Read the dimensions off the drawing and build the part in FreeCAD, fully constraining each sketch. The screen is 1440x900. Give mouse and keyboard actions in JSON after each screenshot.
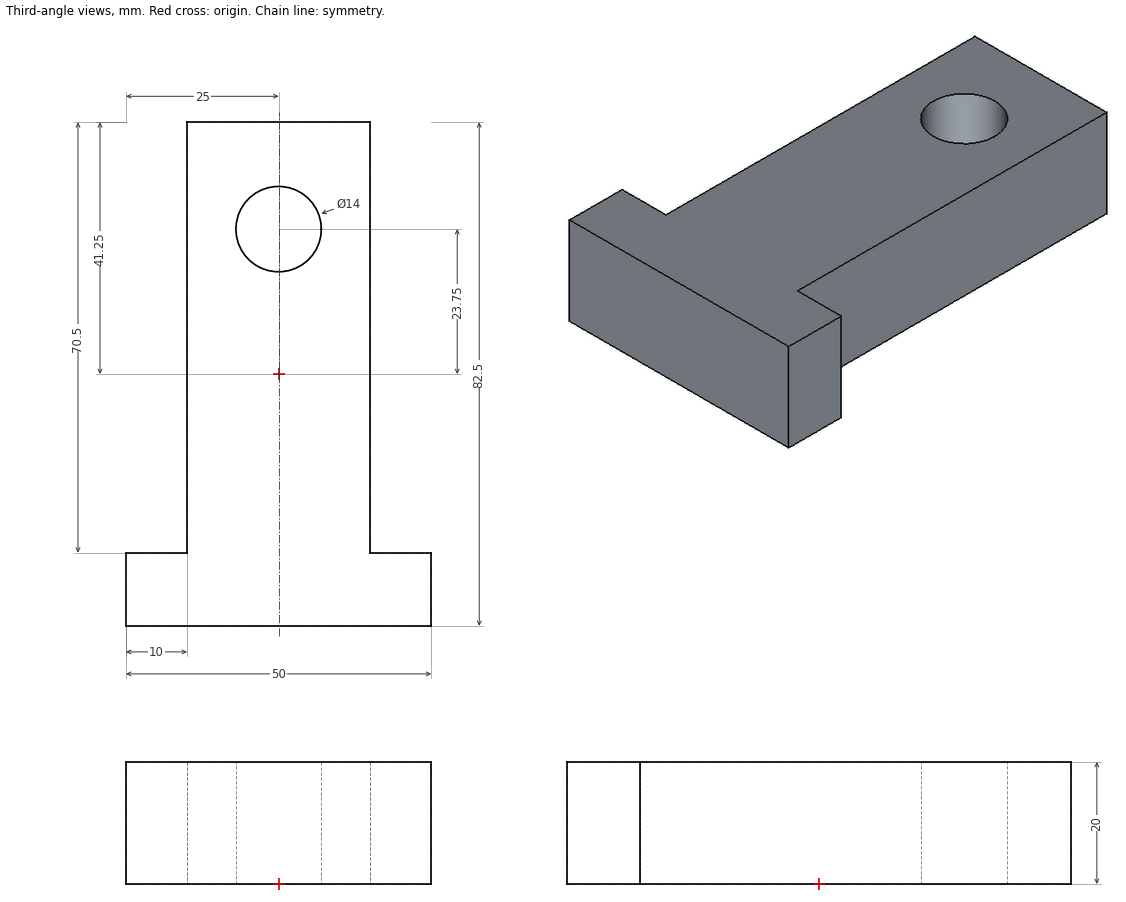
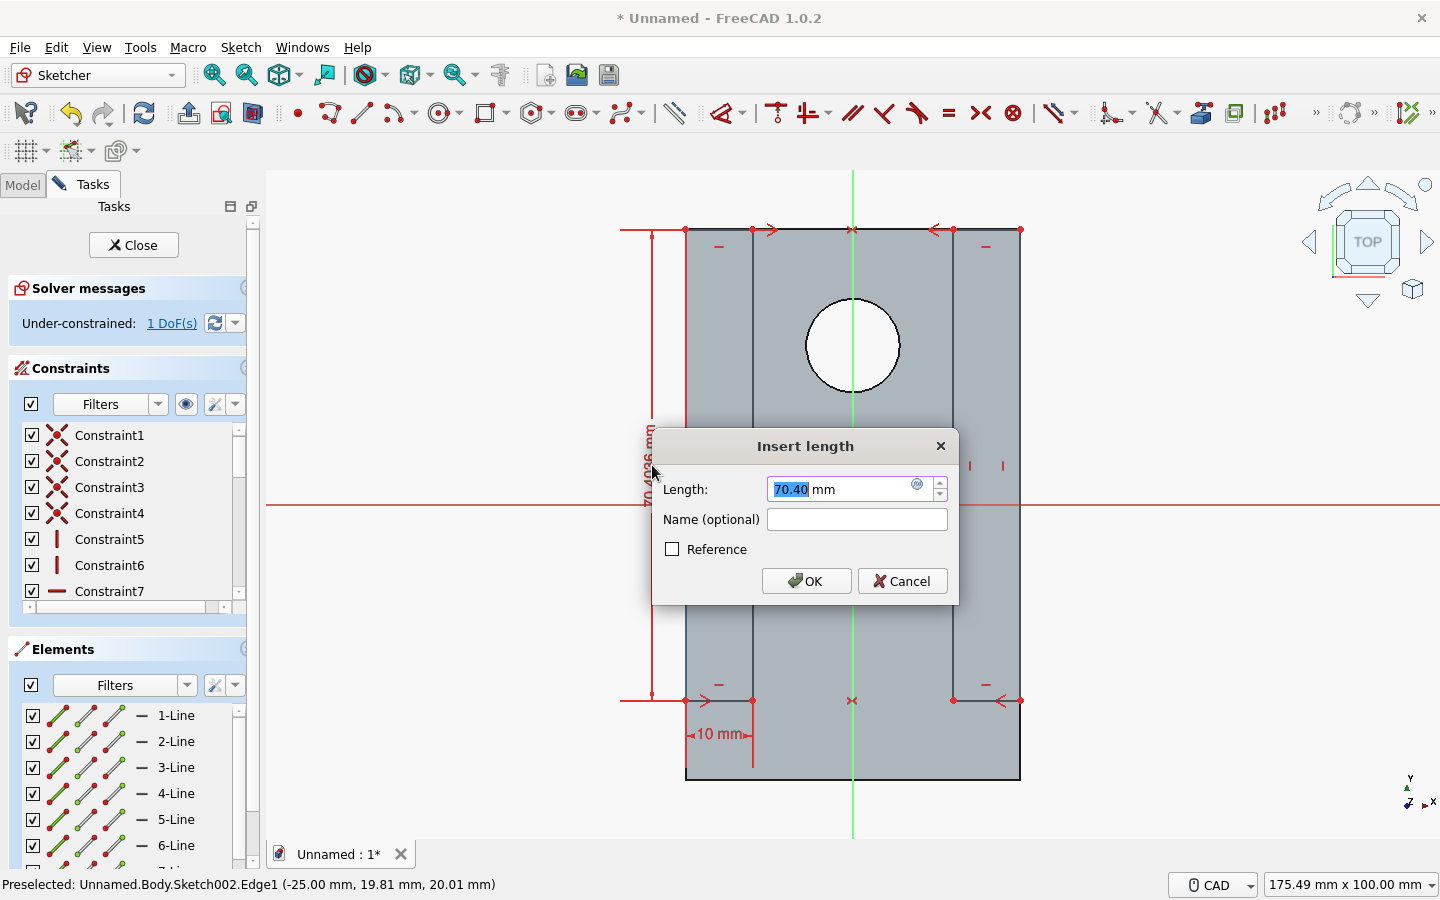
{"action": "type", "text": "70.5"}
{"action": "key", "text": "Return"}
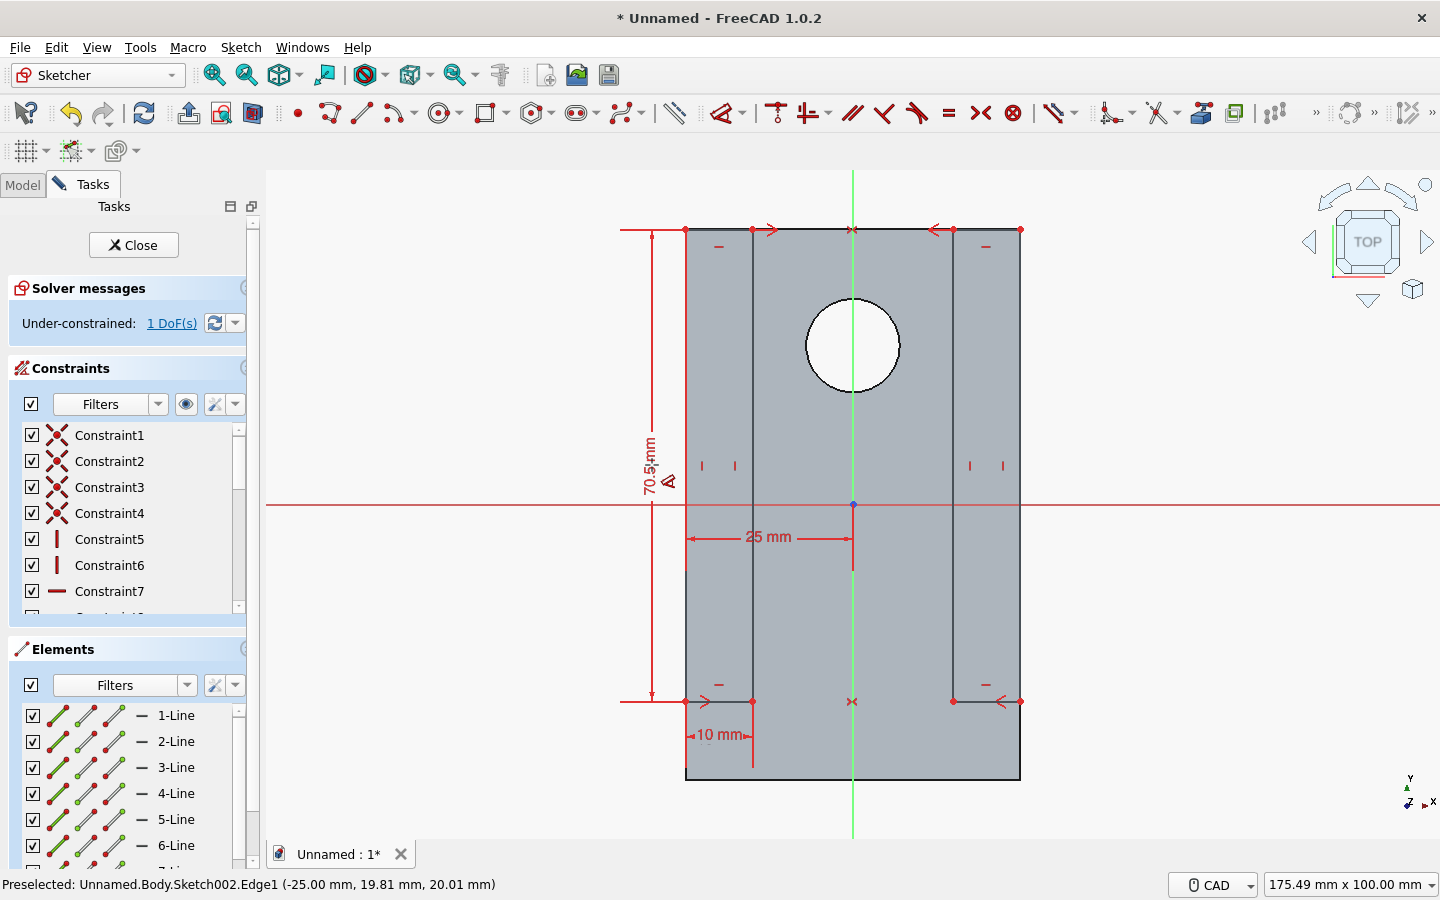
{"action": "left_click", "coordinate": [686, 230]}
{"action": "left_click", "coordinate": [652, 367]}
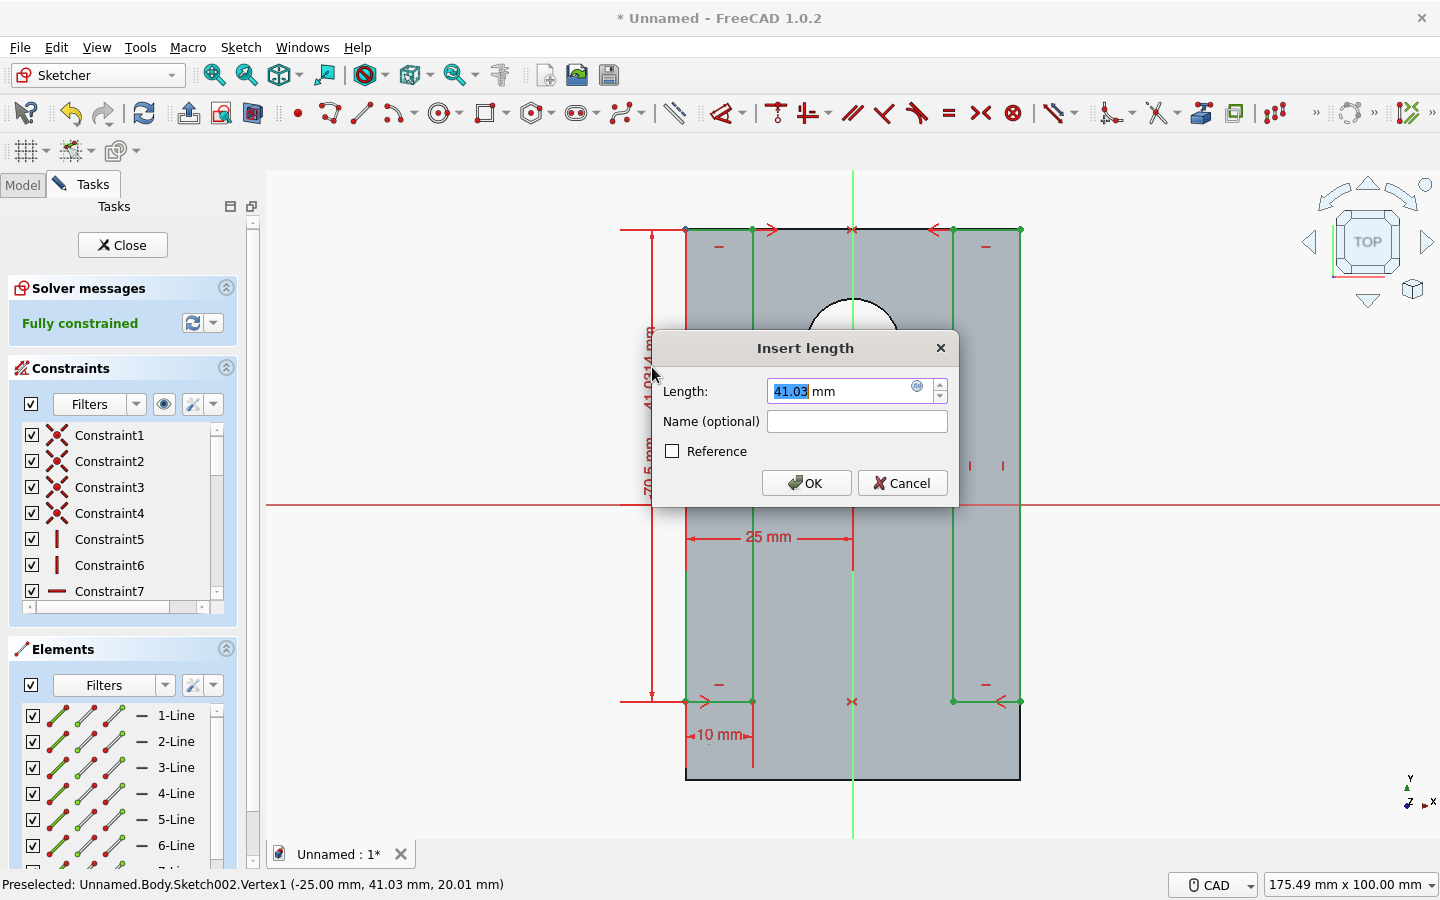
{"action": "type", "text": "41.25"}
{"action": "key", "text": "Return"}
{"action": "key", "text": "Escape"}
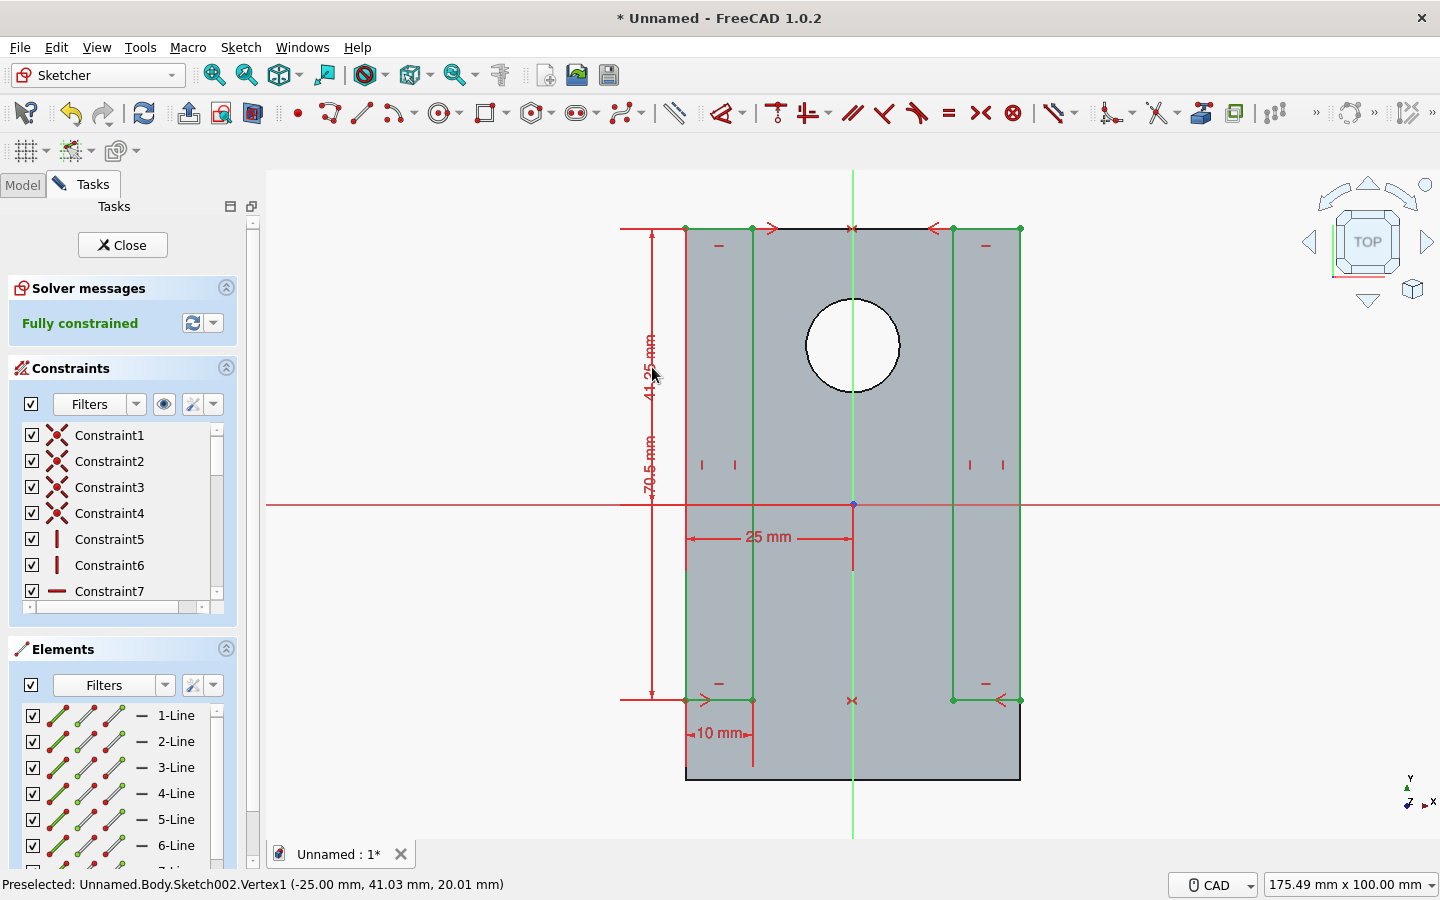
{"action": "left_click", "coordinate": [123, 245]}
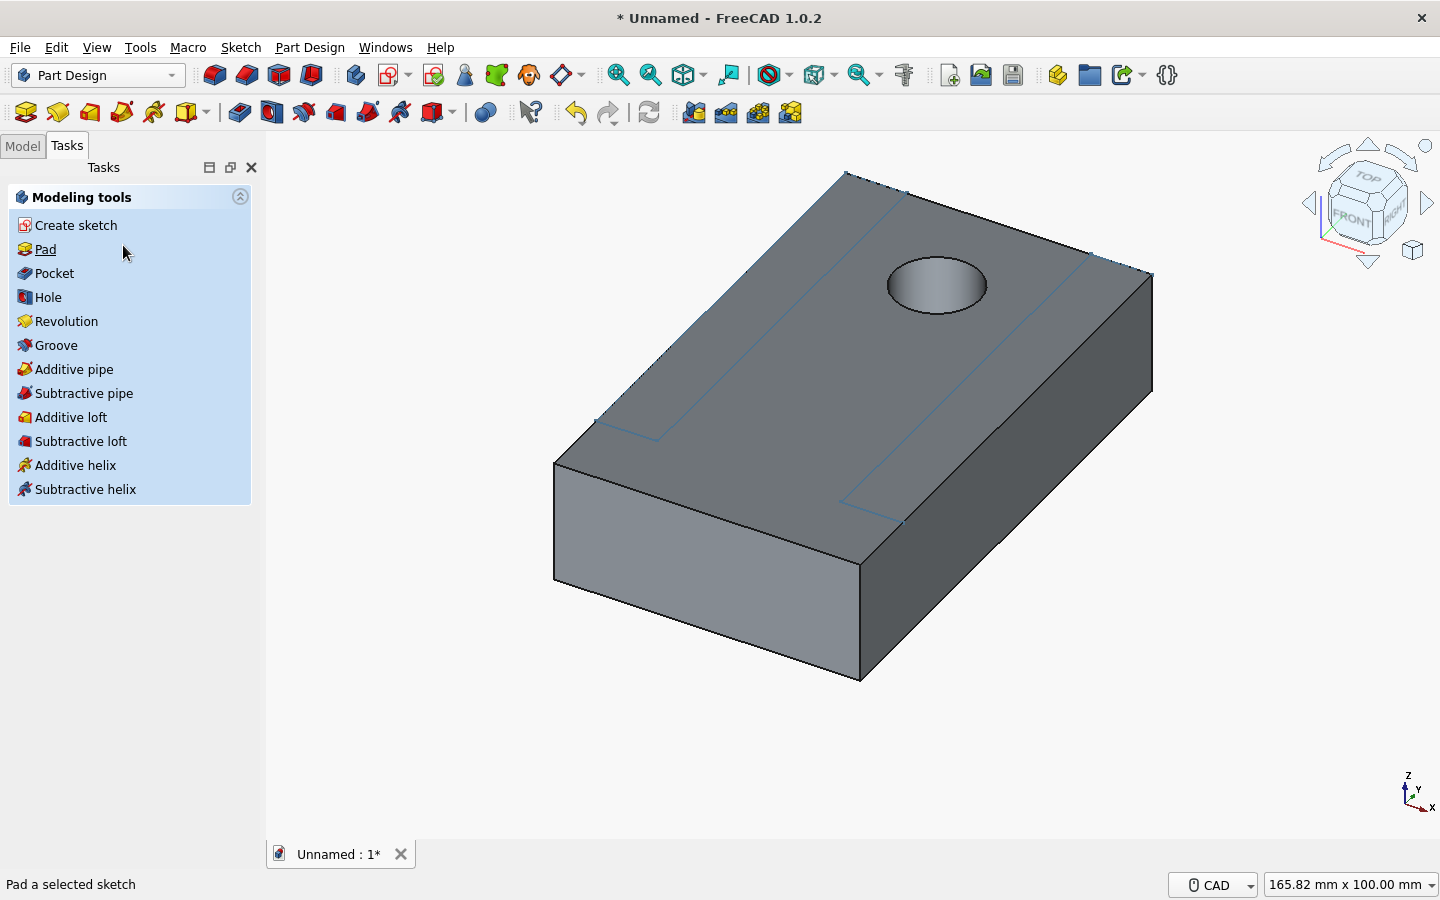
{"action": "left_click", "coordinate": [240, 112]}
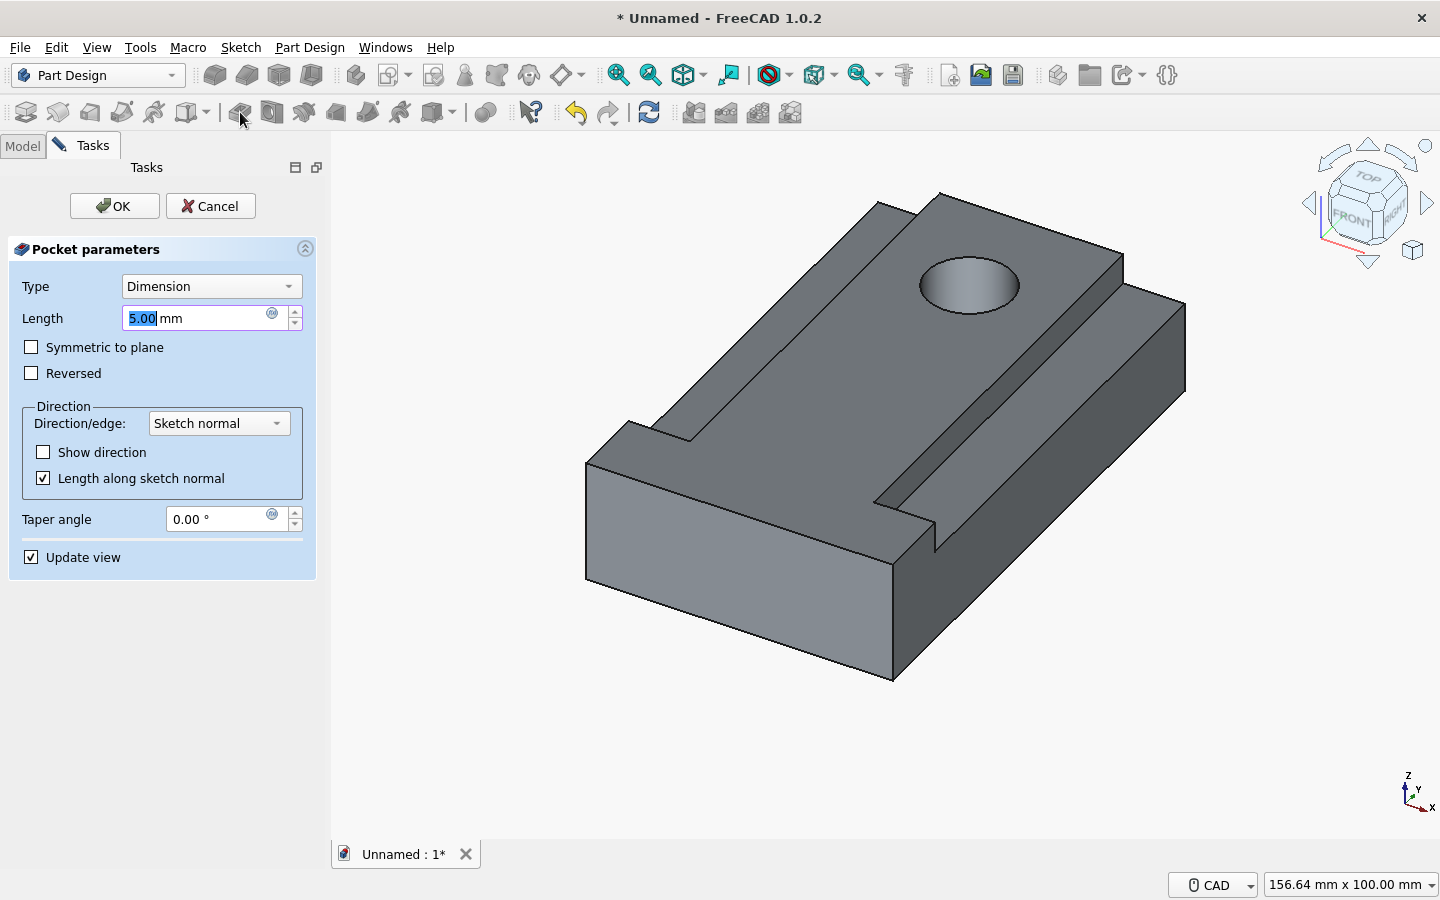
{"action": "left_click", "coordinate": [212, 286]}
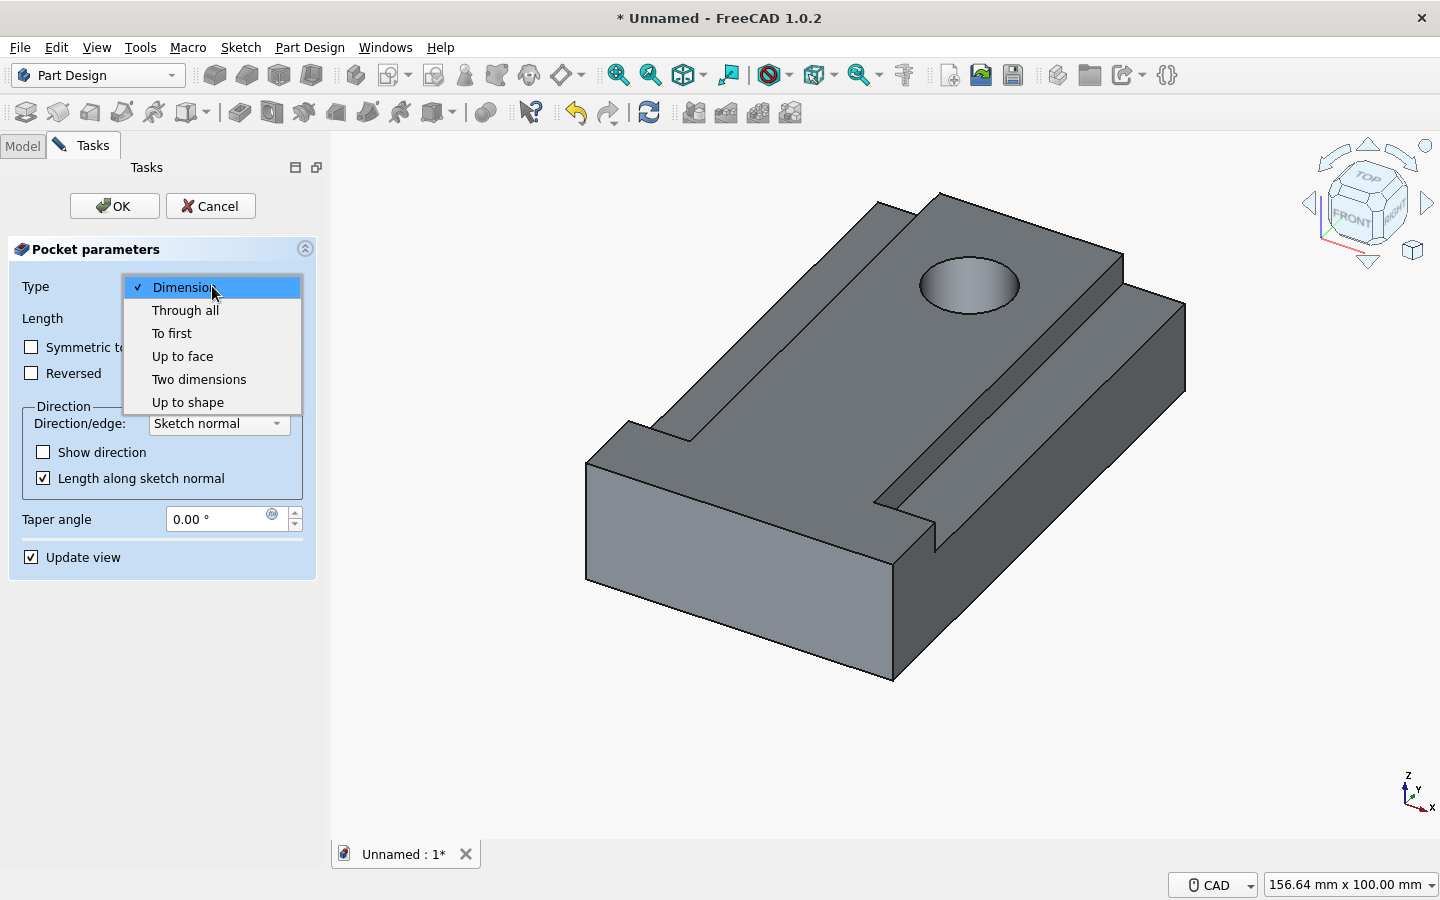
{"action": "left_click", "coordinate": [212, 310]}